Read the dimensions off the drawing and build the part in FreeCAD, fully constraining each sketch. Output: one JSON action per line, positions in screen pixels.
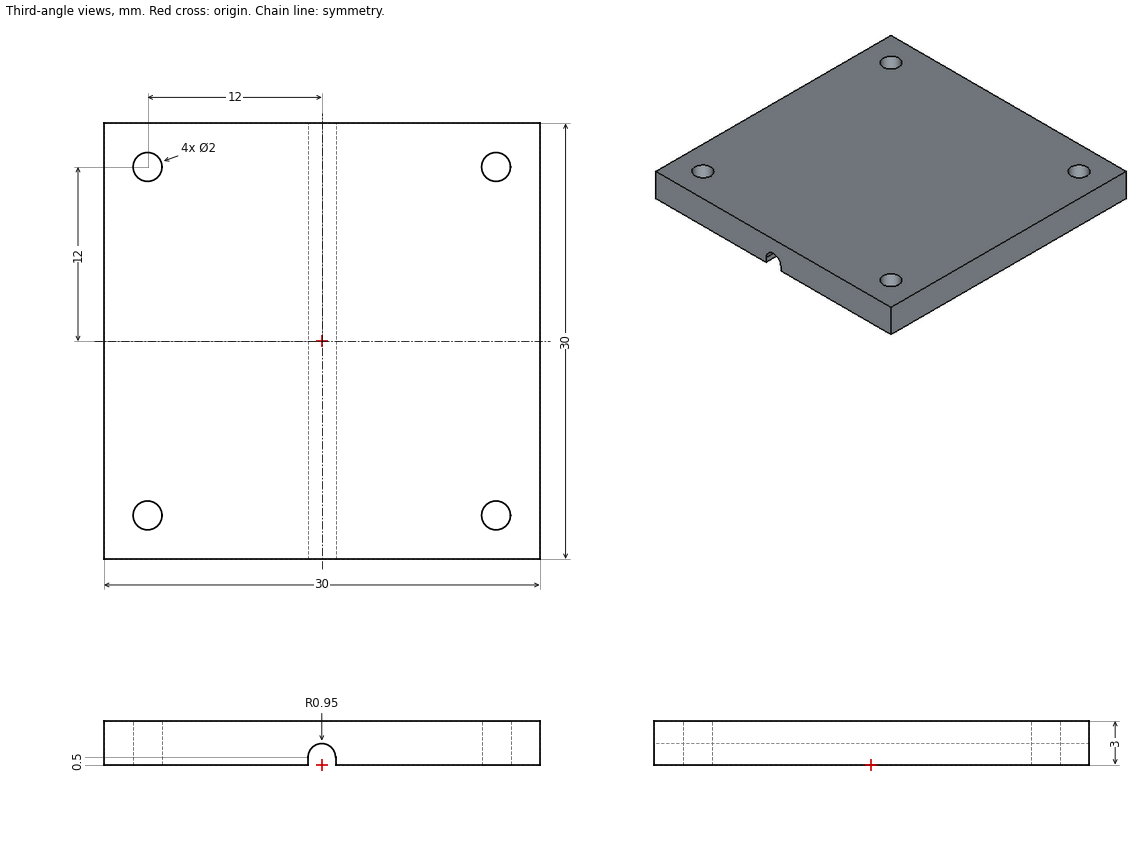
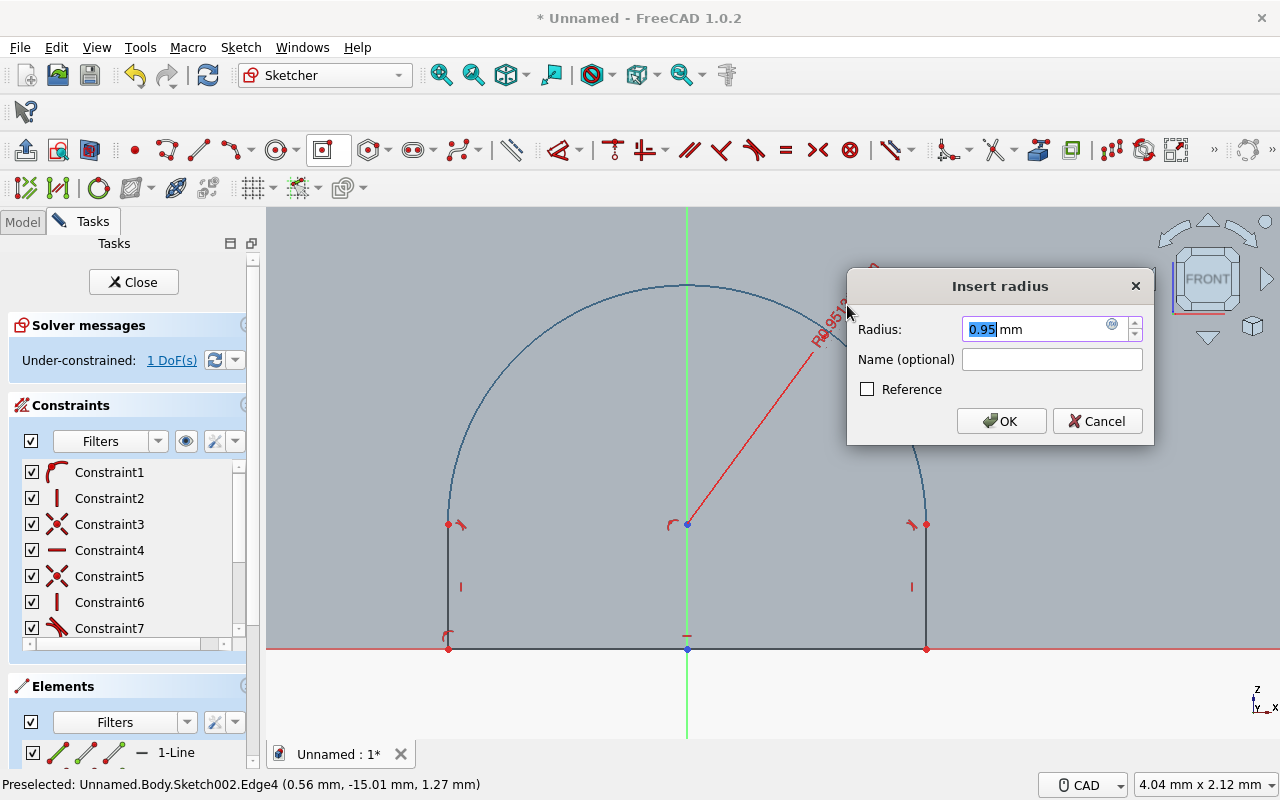
{"action": "type", "text": "0.95"}
{"action": "key", "text": "Return"}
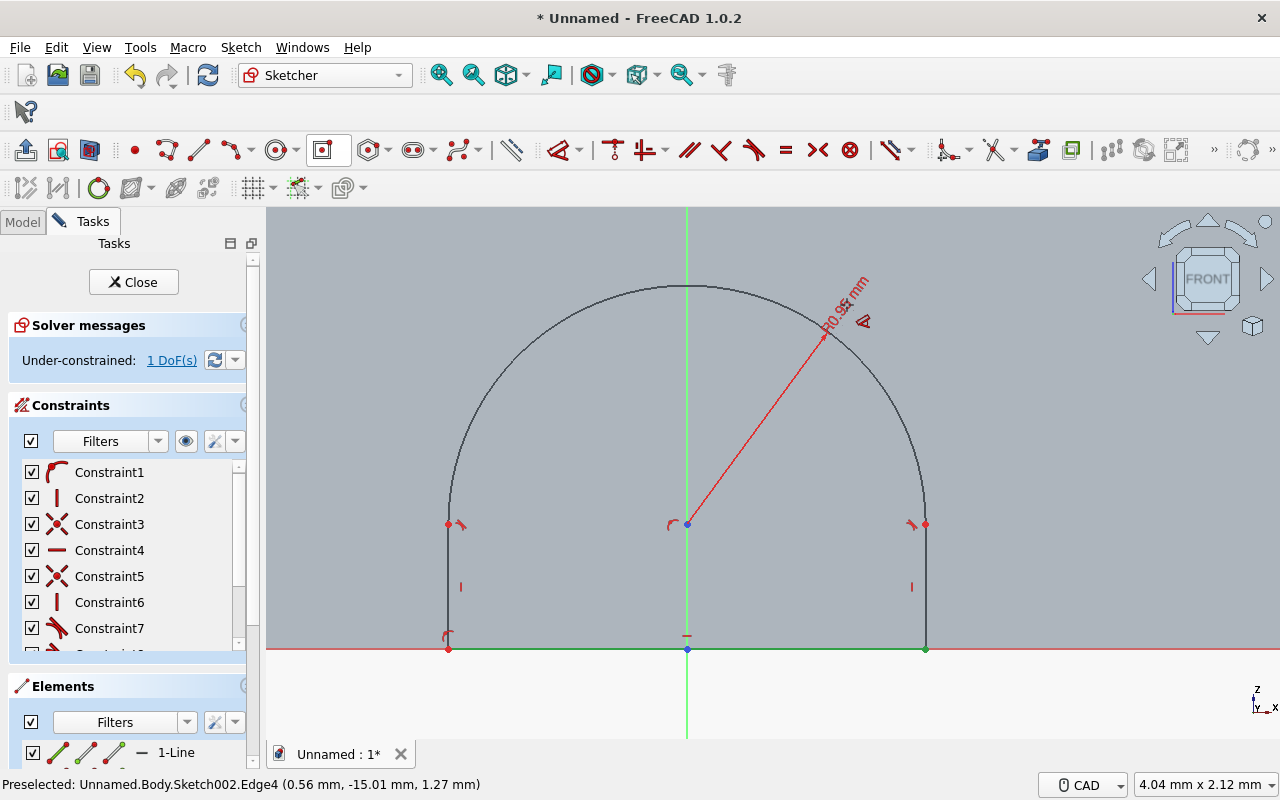
{"action": "left_click", "coordinate": [448, 562]}
{"action": "left_click", "coordinate": [414, 587]}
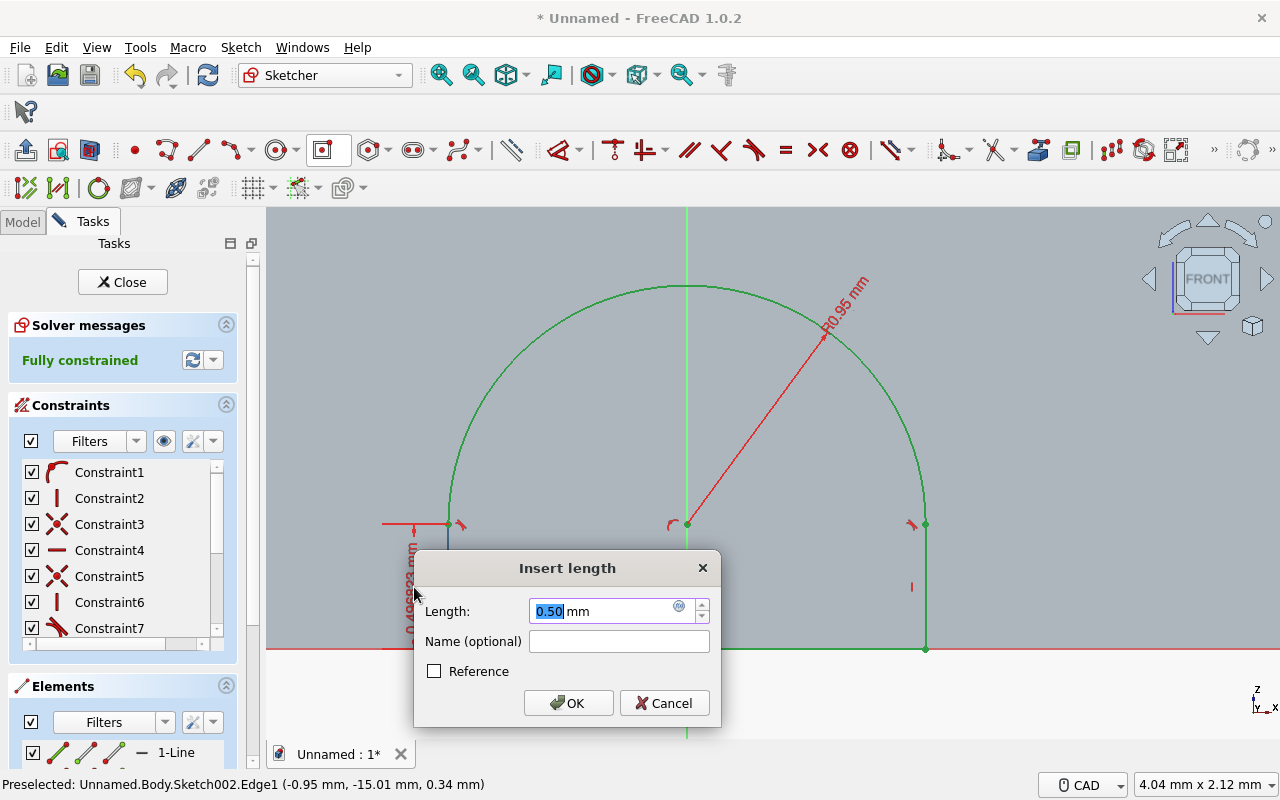
{"action": "type", "text": "0.5"}
{"action": "key", "text": "Return"}
{"action": "key", "text": "Escape"}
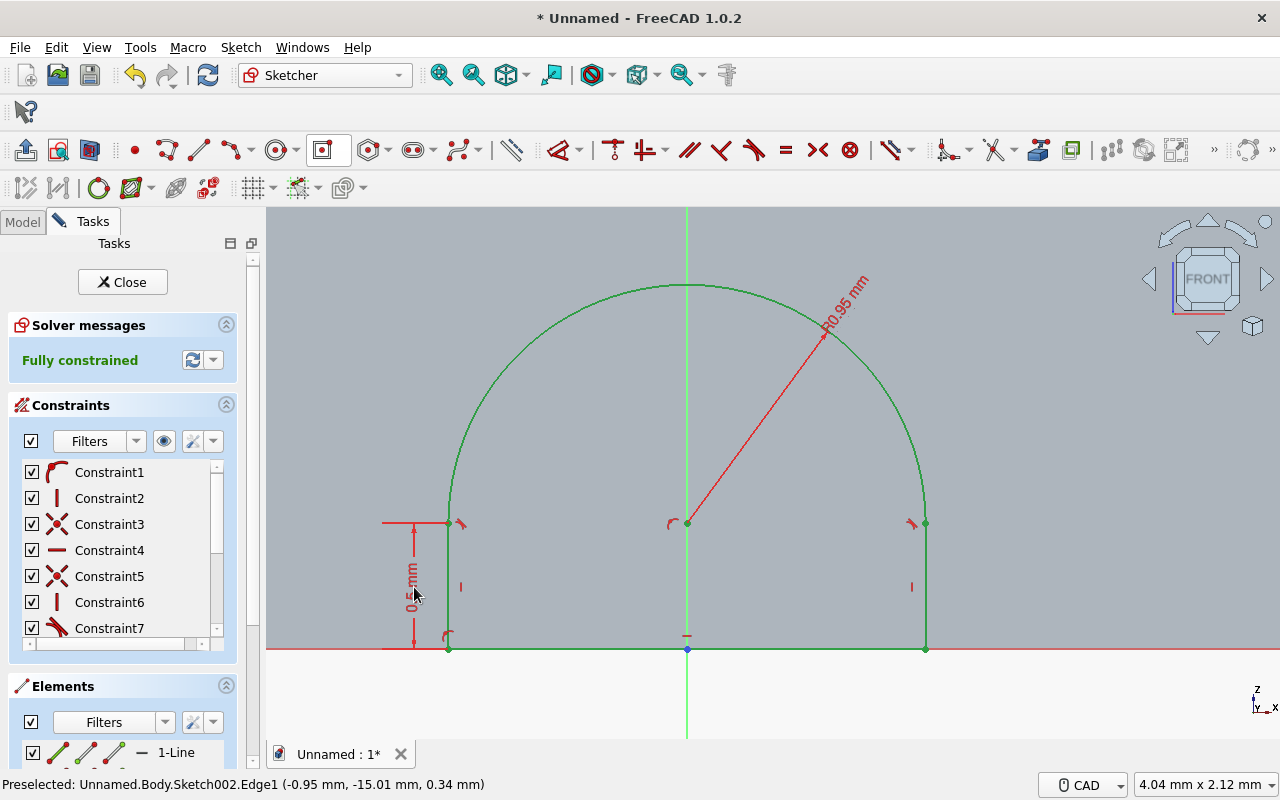
{"action": "left_click", "coordinate": [123, 282]}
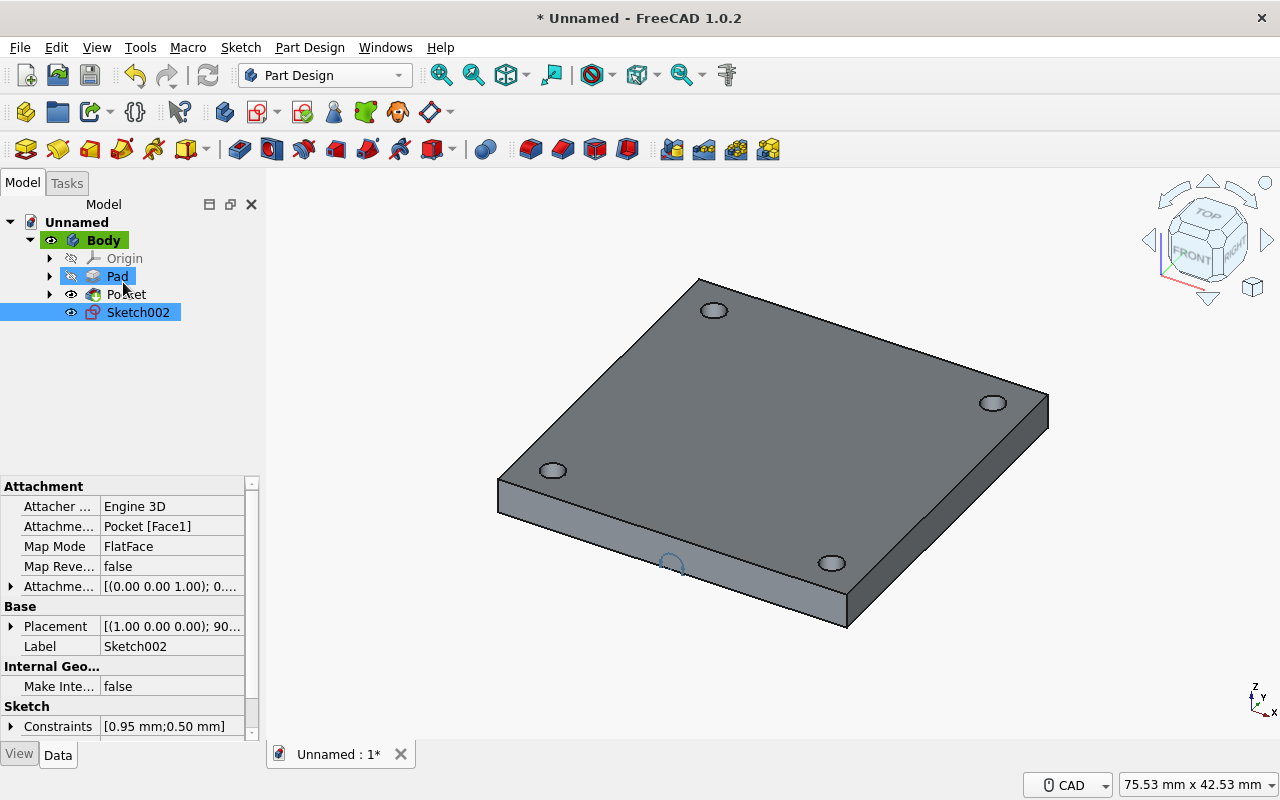
{"action": "left_click", "coordinate": [240, 150]}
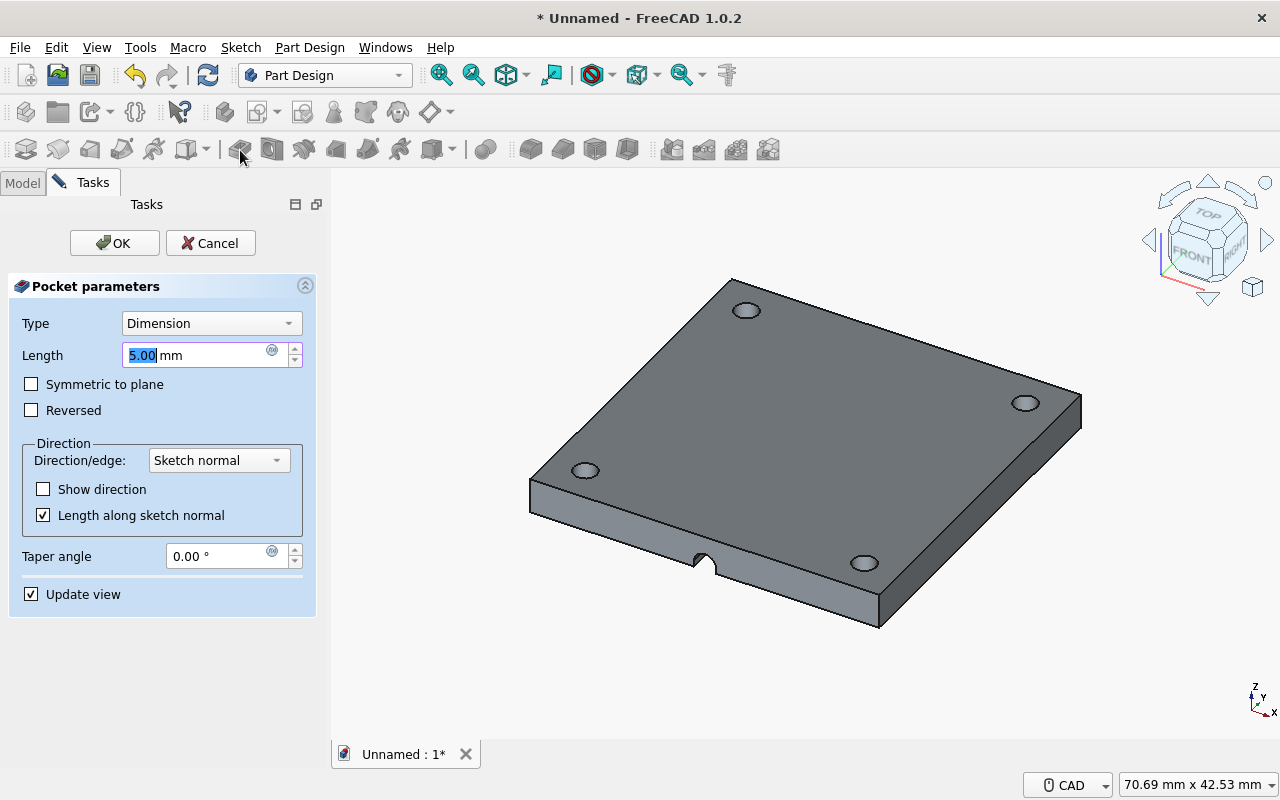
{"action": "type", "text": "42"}
{"action": "key", "text": "Tab"}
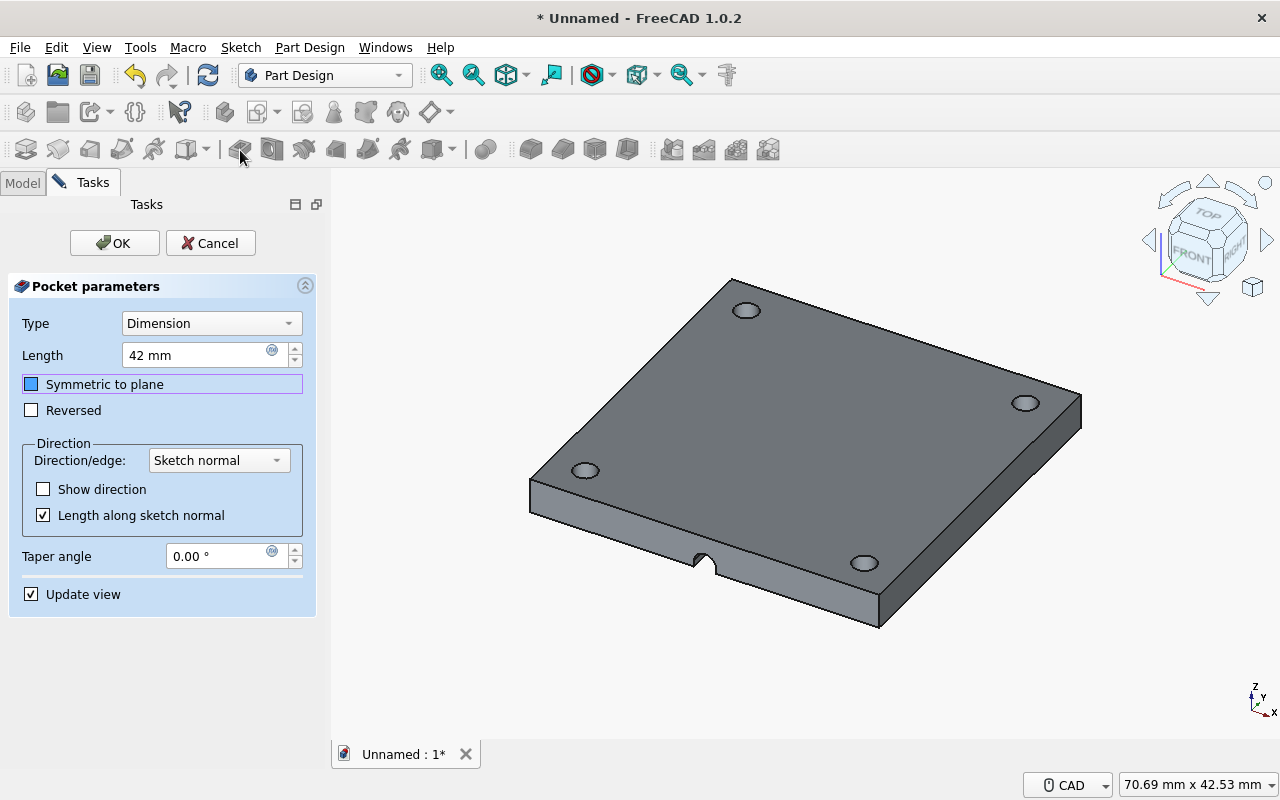
{"action": "left_click", "coordinate": [115, 243]}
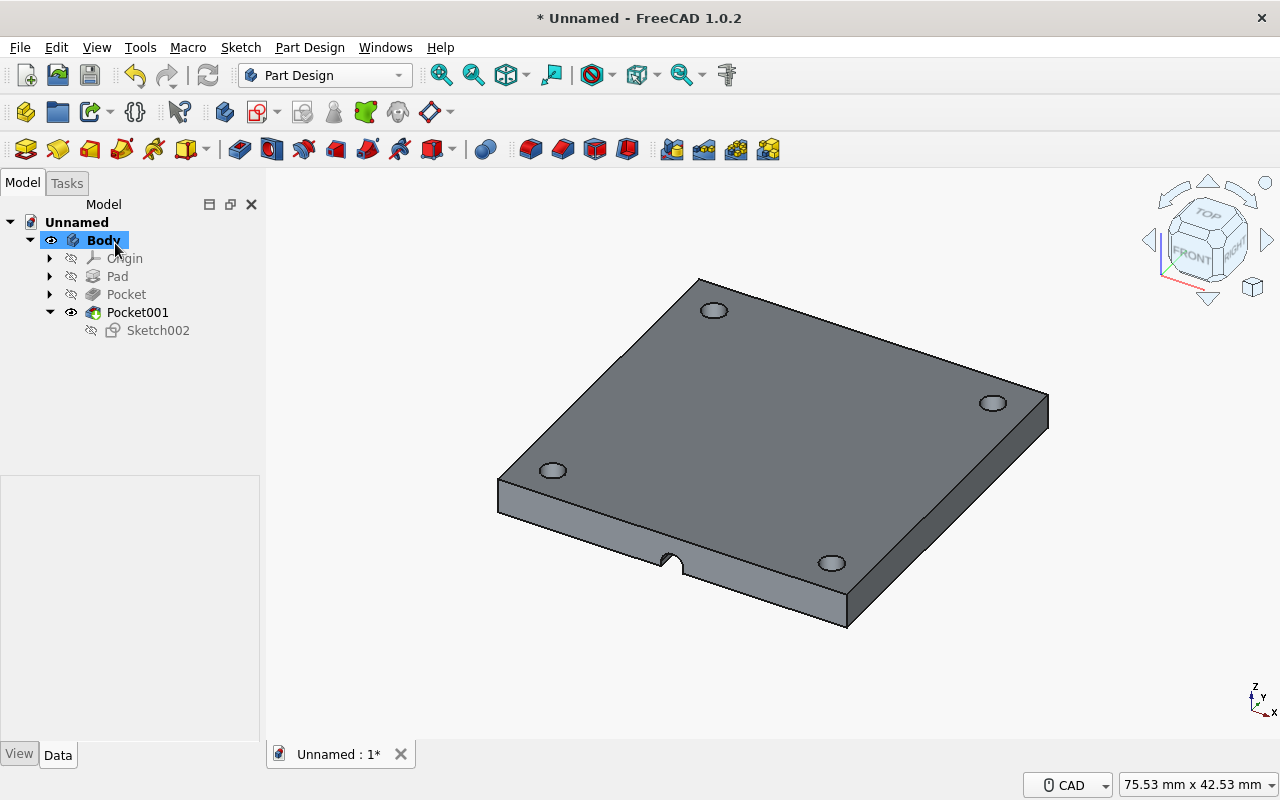
{"action": "key", "text": "0"}